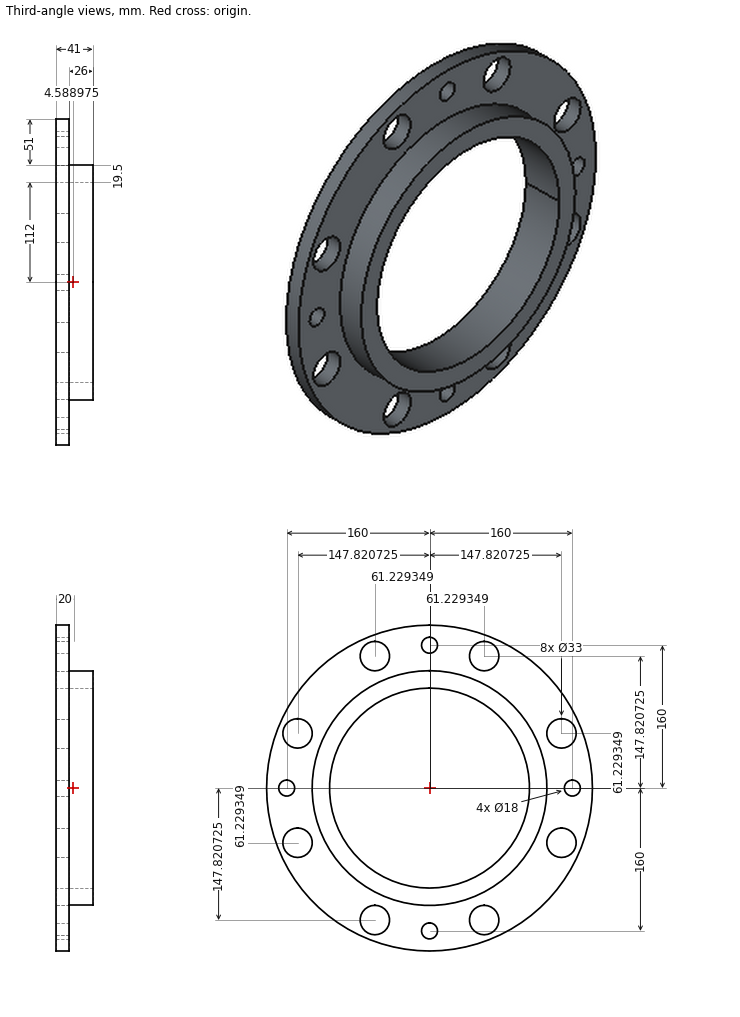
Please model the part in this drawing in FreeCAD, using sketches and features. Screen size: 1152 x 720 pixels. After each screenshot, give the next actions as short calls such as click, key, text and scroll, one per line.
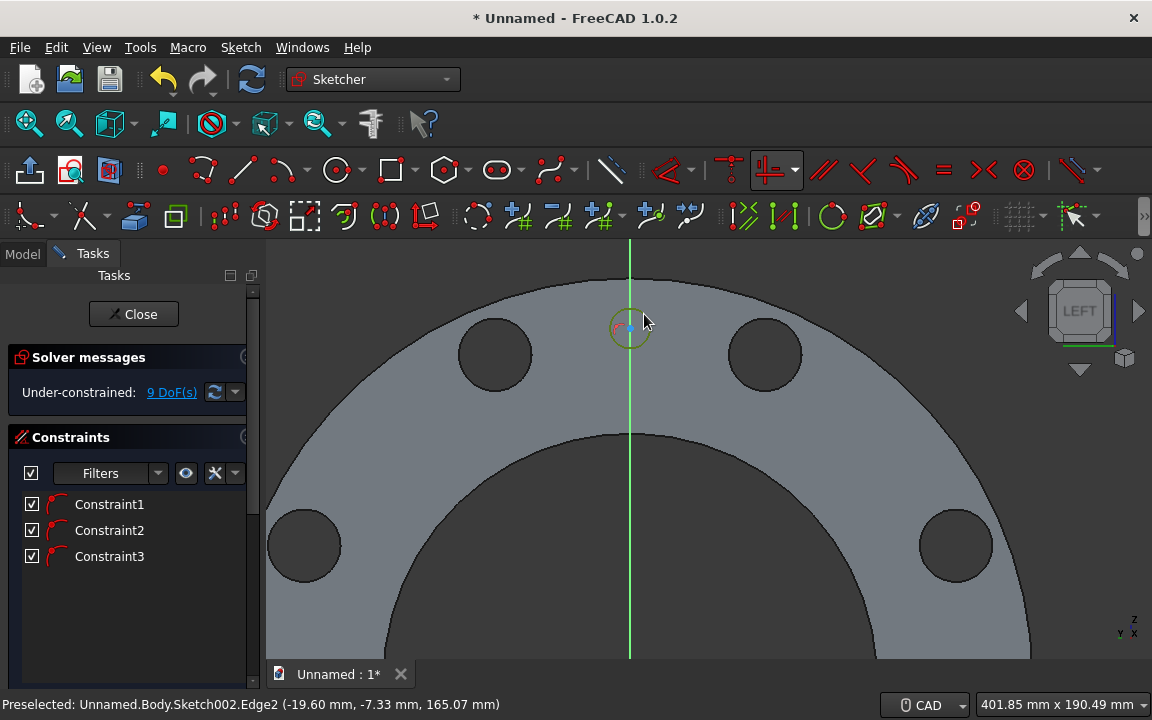
scroll(647, 314, down, 5)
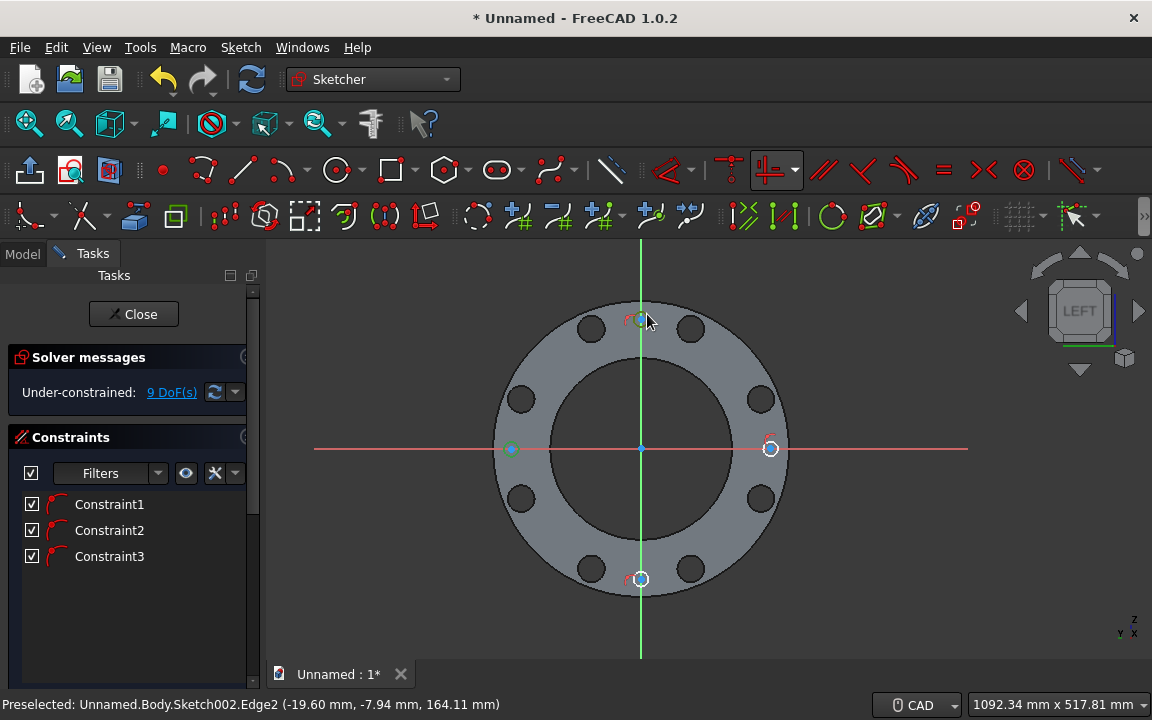
scroll(776, 444, up, 5)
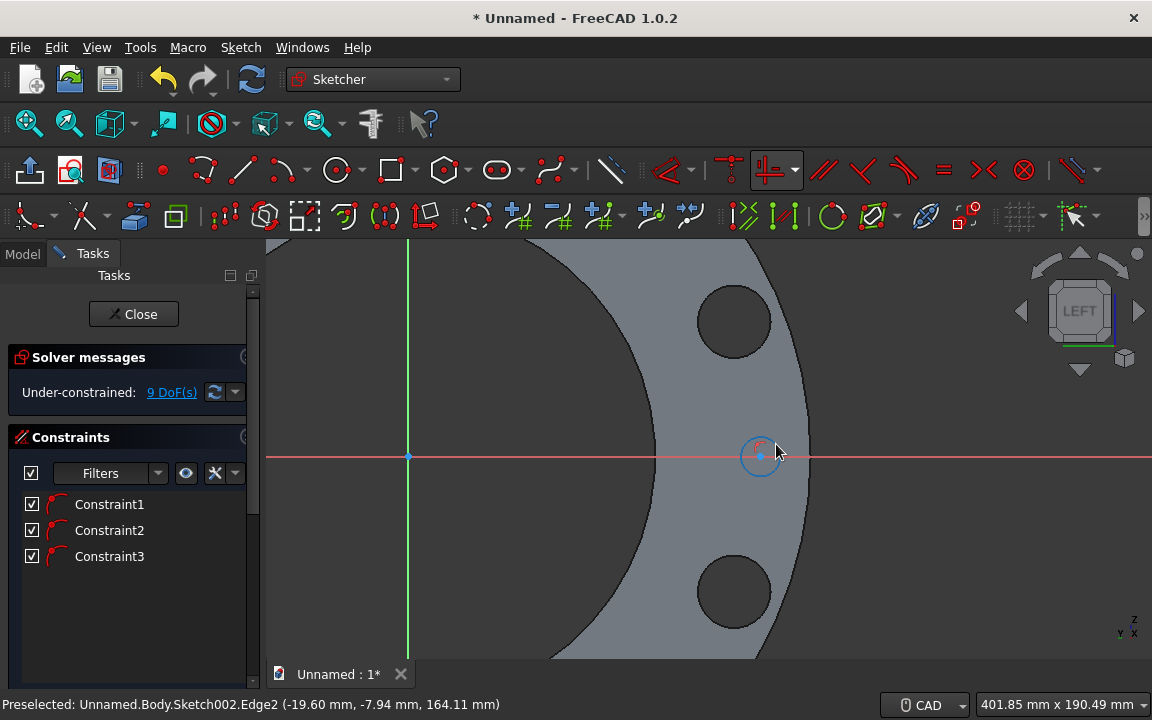
click(775, 443)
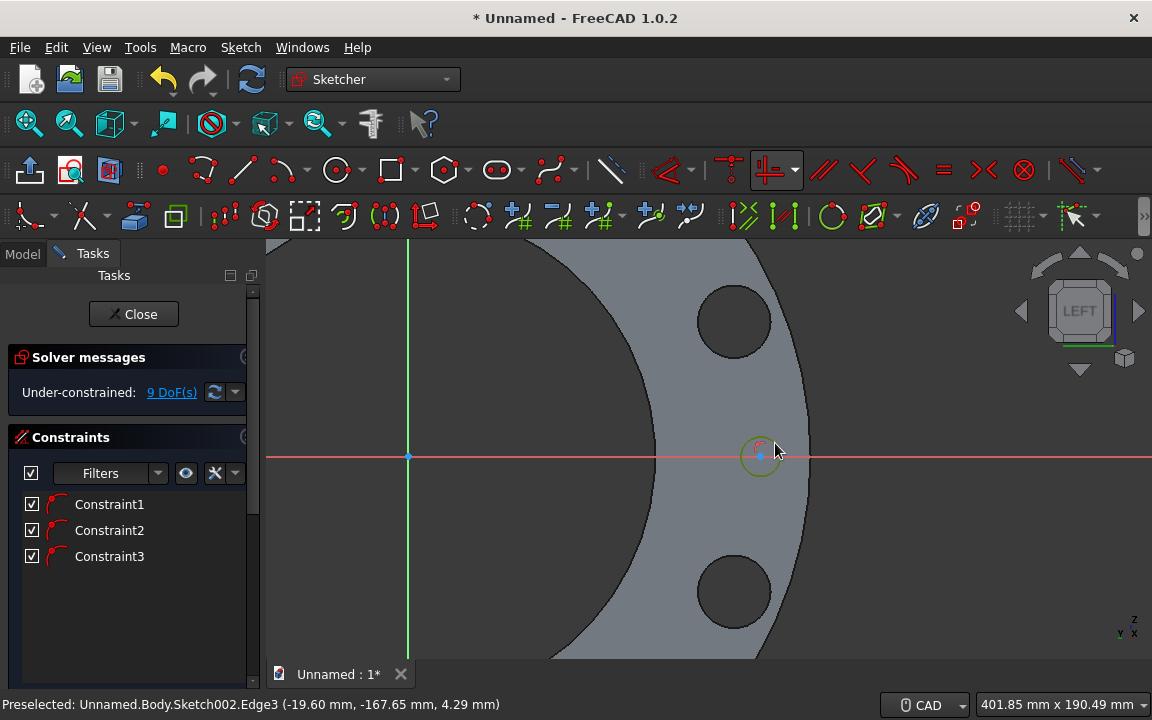
scroll(776, 444, down, 5)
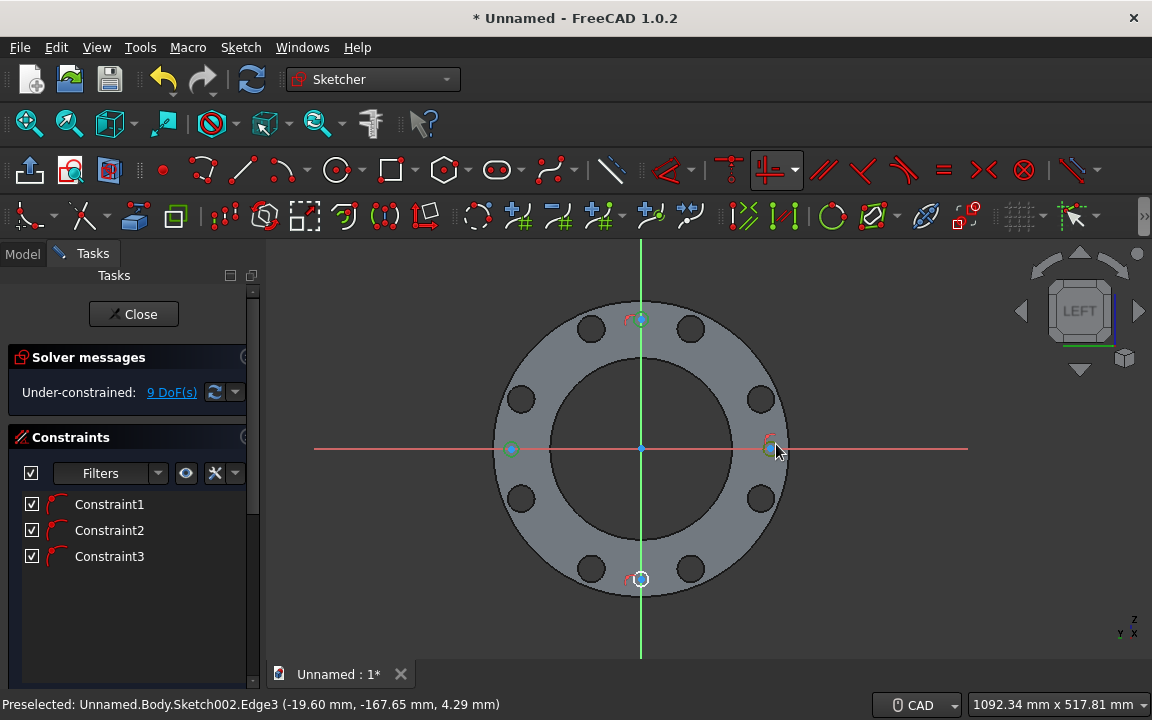
scroll(646, 574, up, 5)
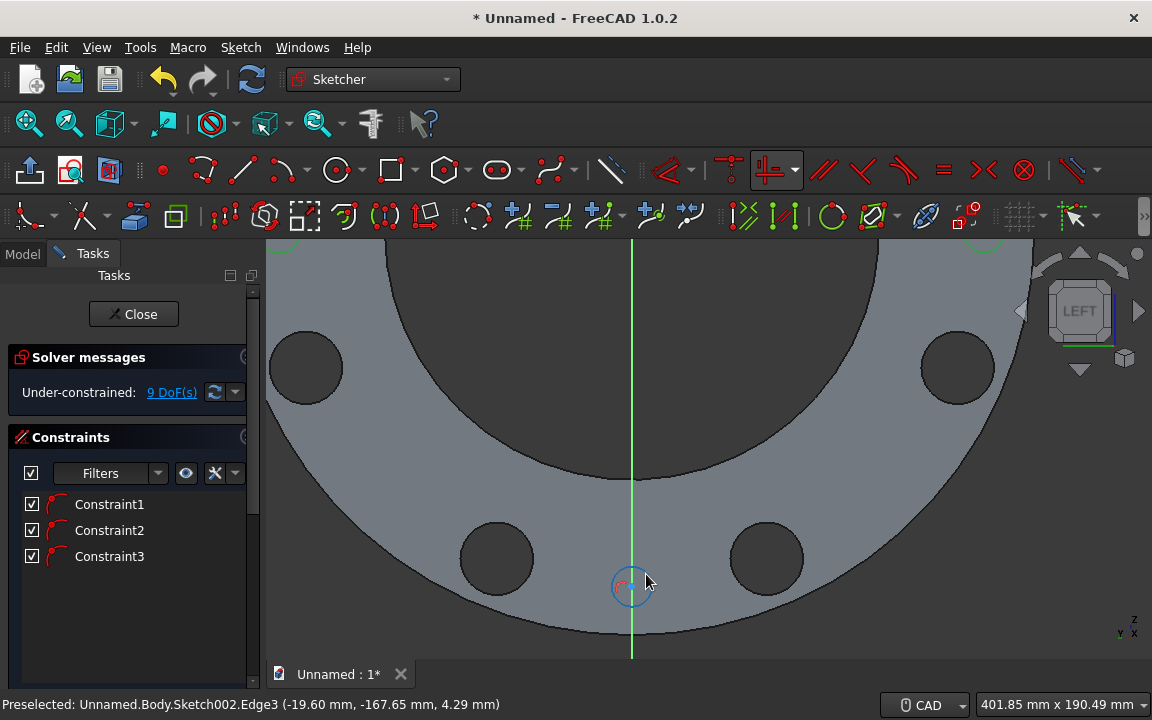
click(646, 572)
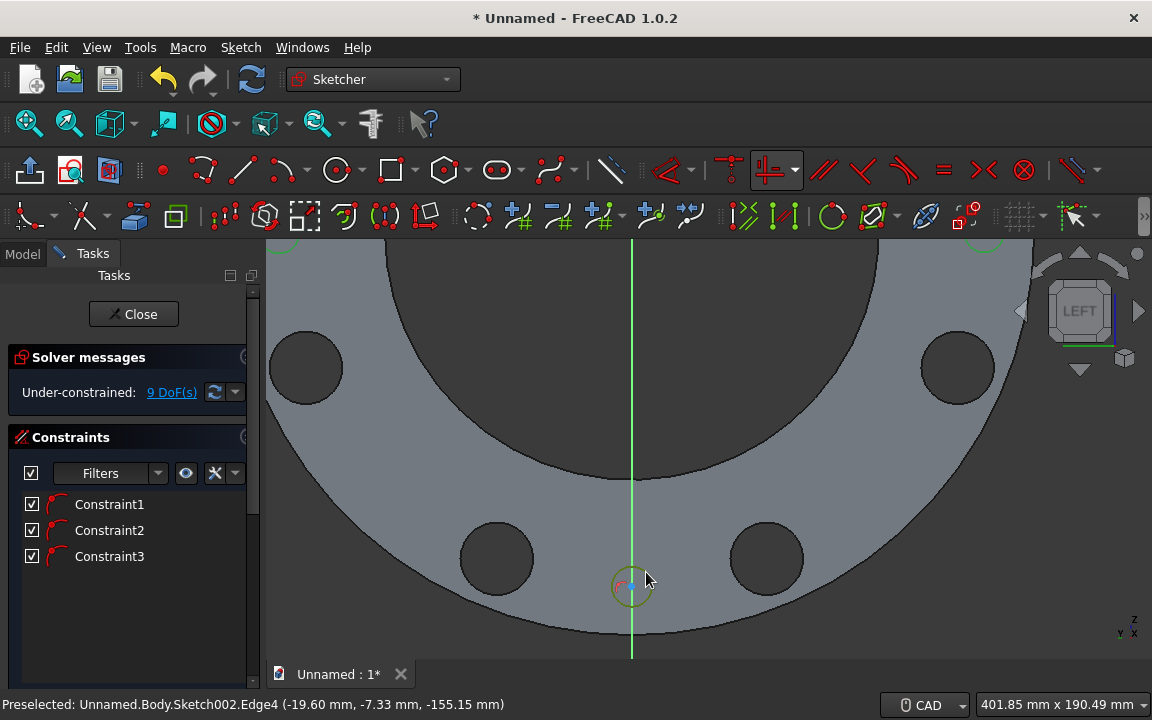
key(e)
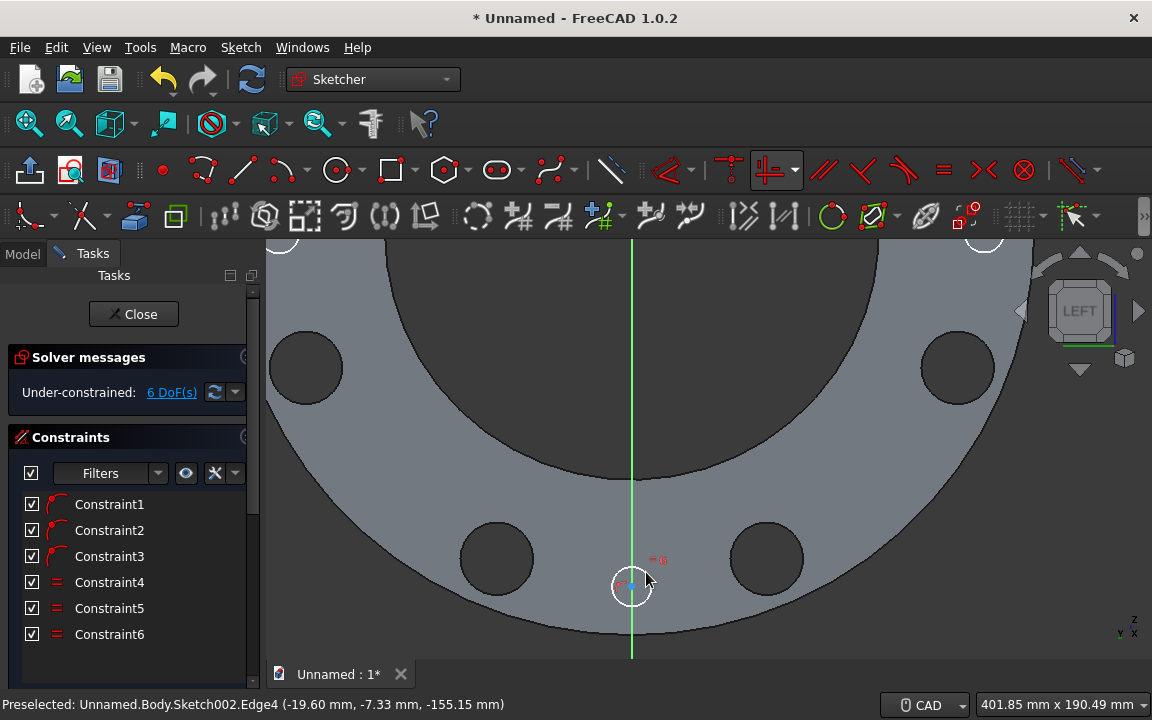
scroll(646, 575, down, 5)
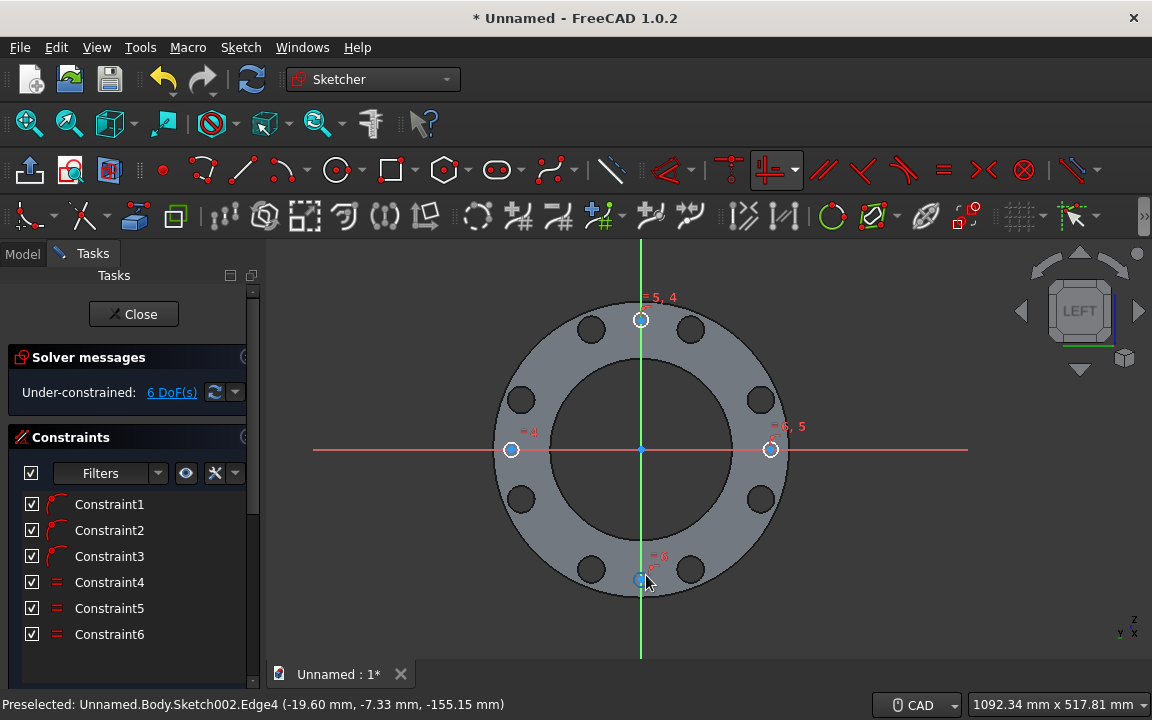
click(511, 450)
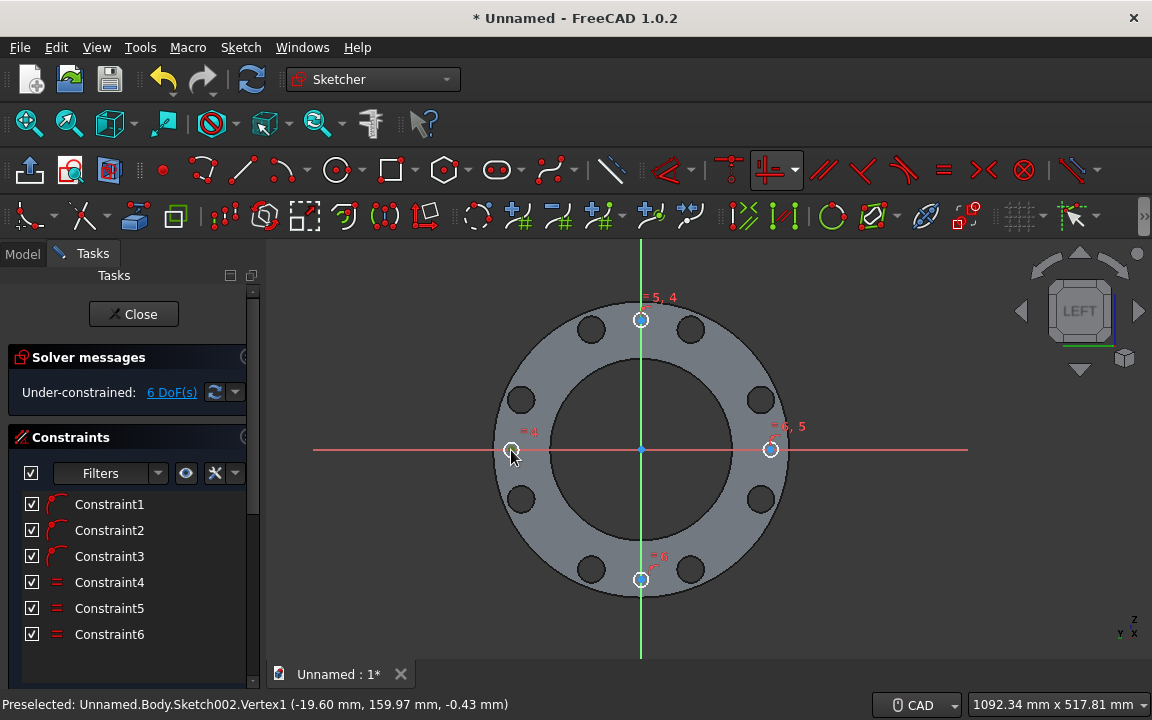
click(344, 450)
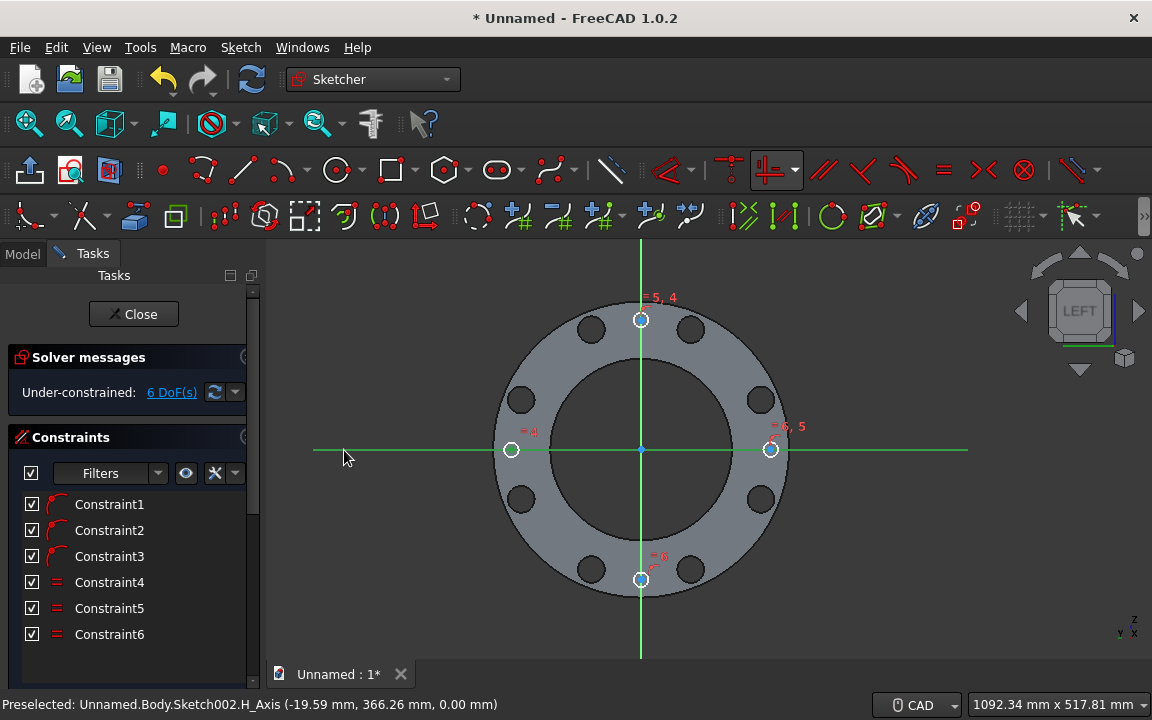
click(730, 170)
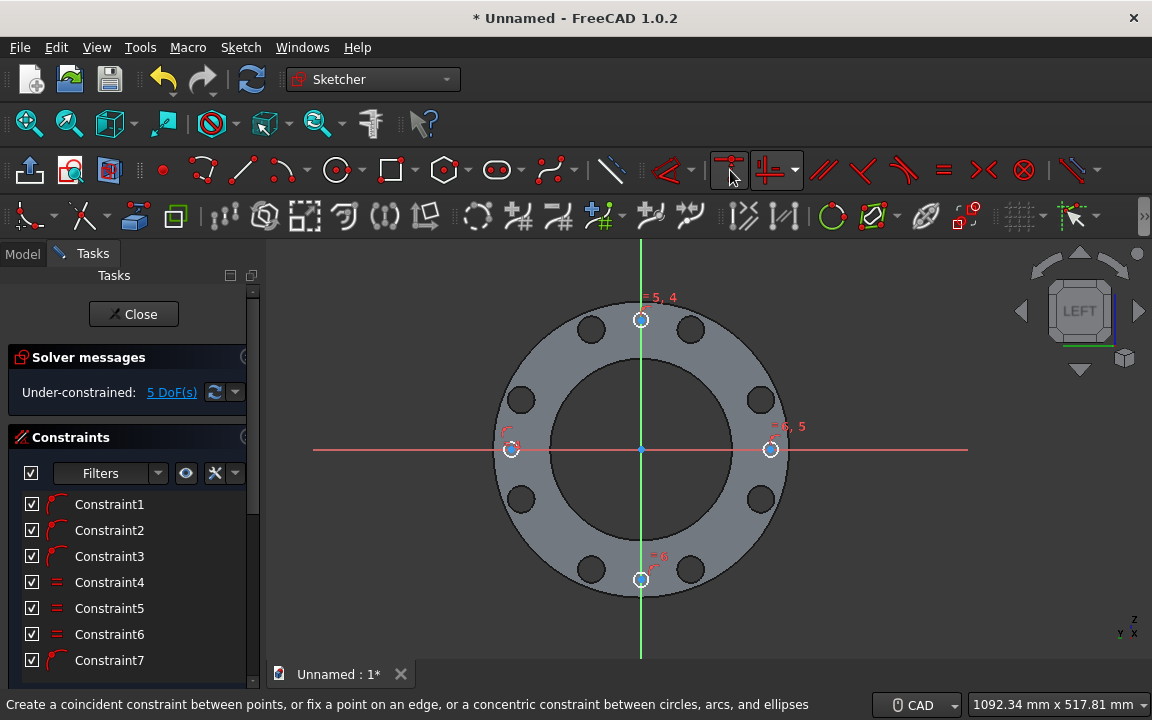
click(666, 170)